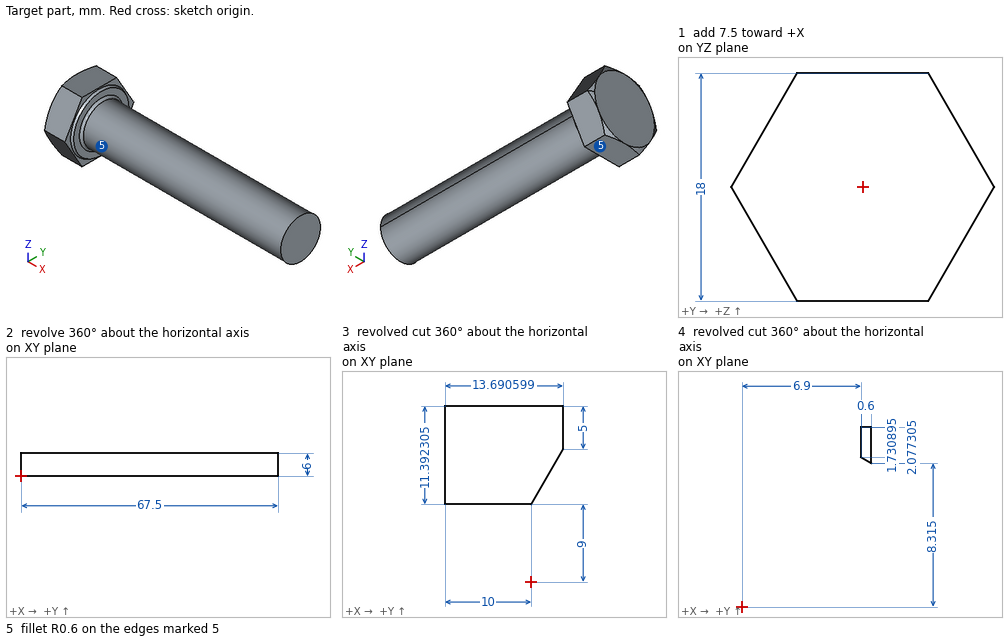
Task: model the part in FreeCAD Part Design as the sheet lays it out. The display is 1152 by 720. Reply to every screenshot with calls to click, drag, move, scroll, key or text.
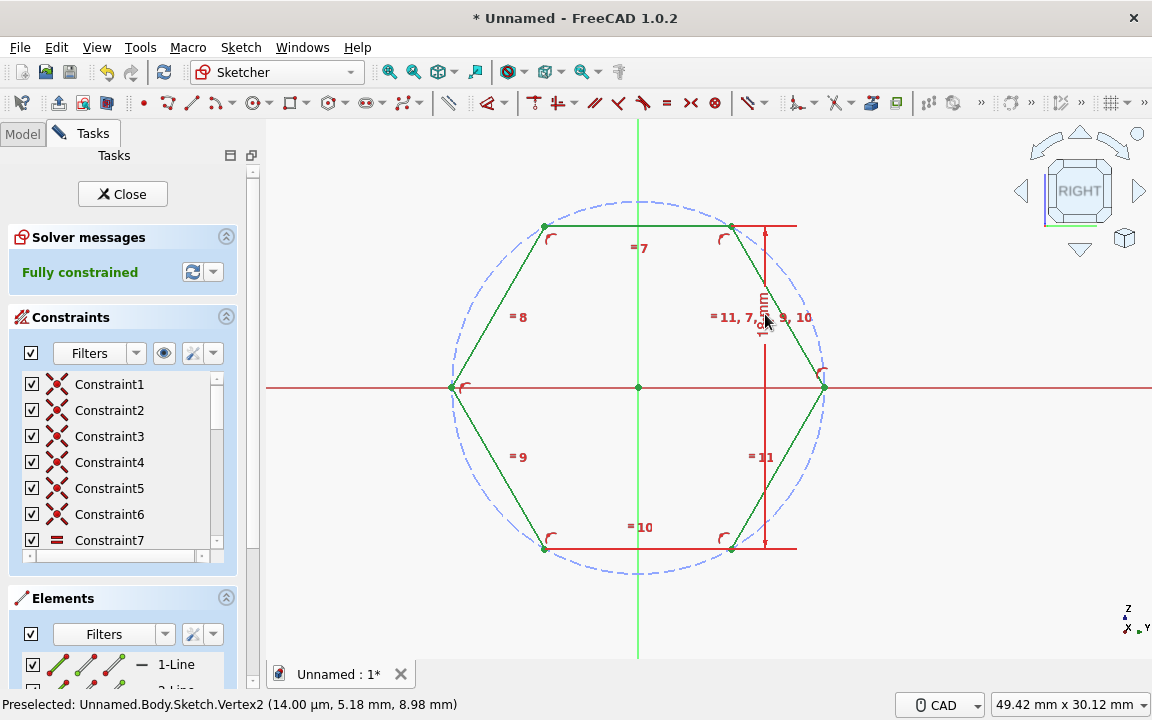
click(123, 194)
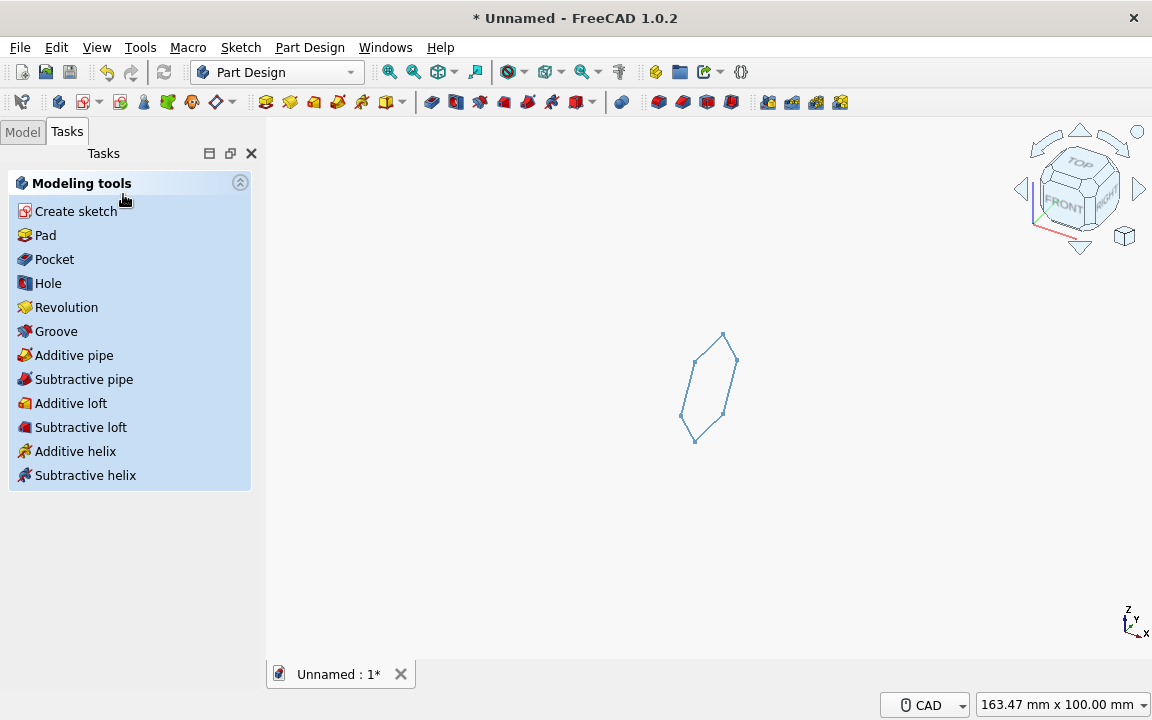
click(266, 102)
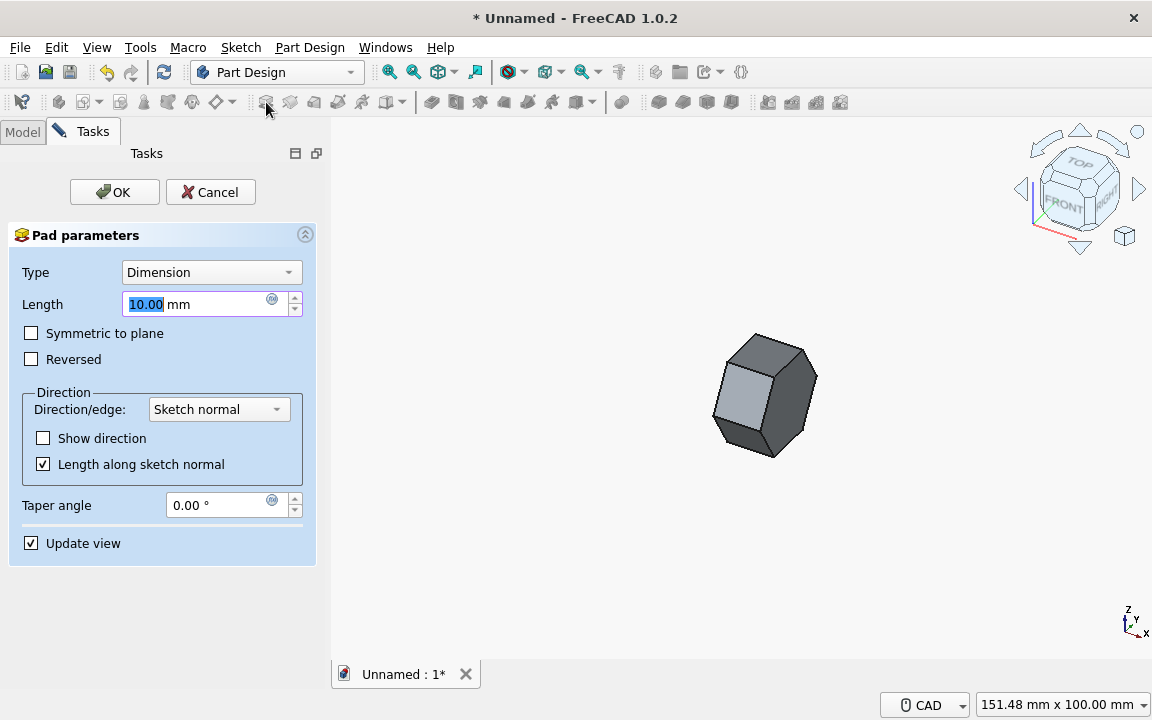
text(7.5)
key(Tab)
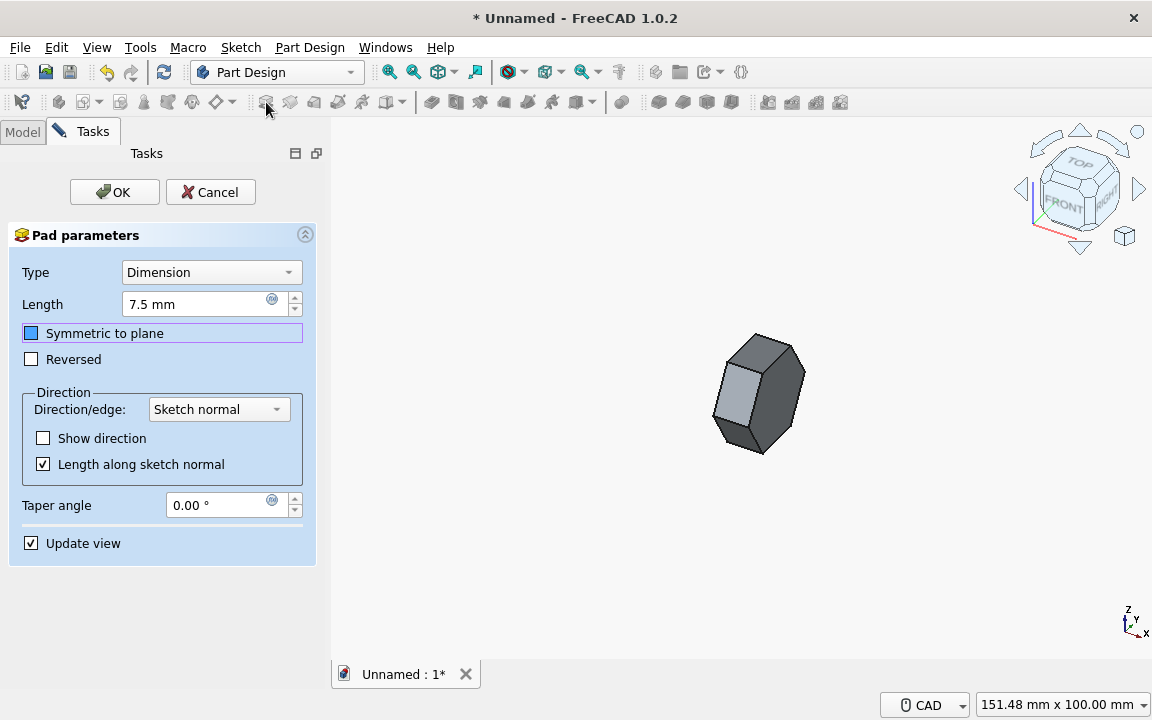
click(115, 192)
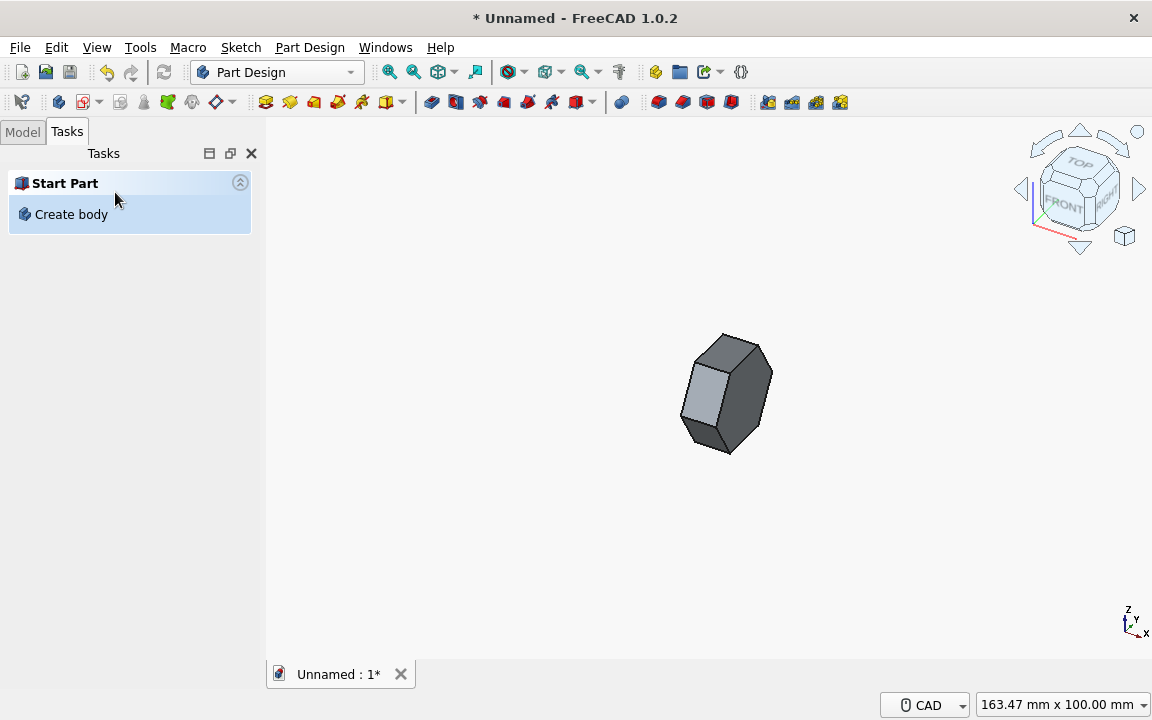
click(390, 72)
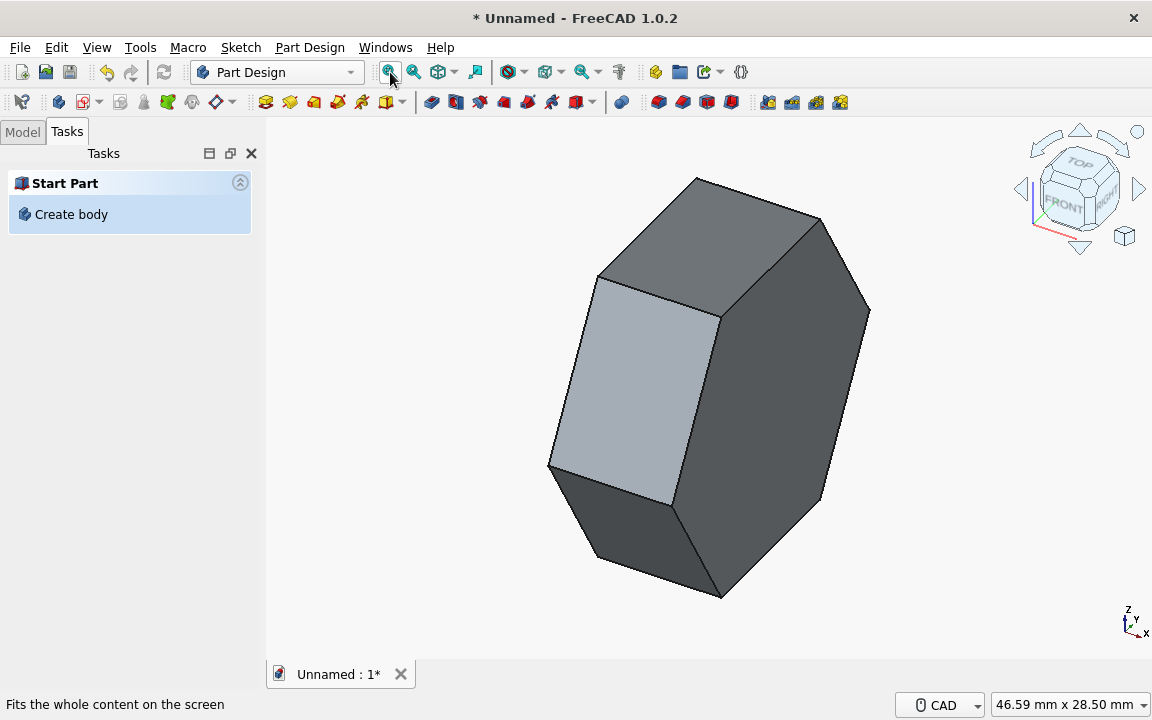
click(84, 102)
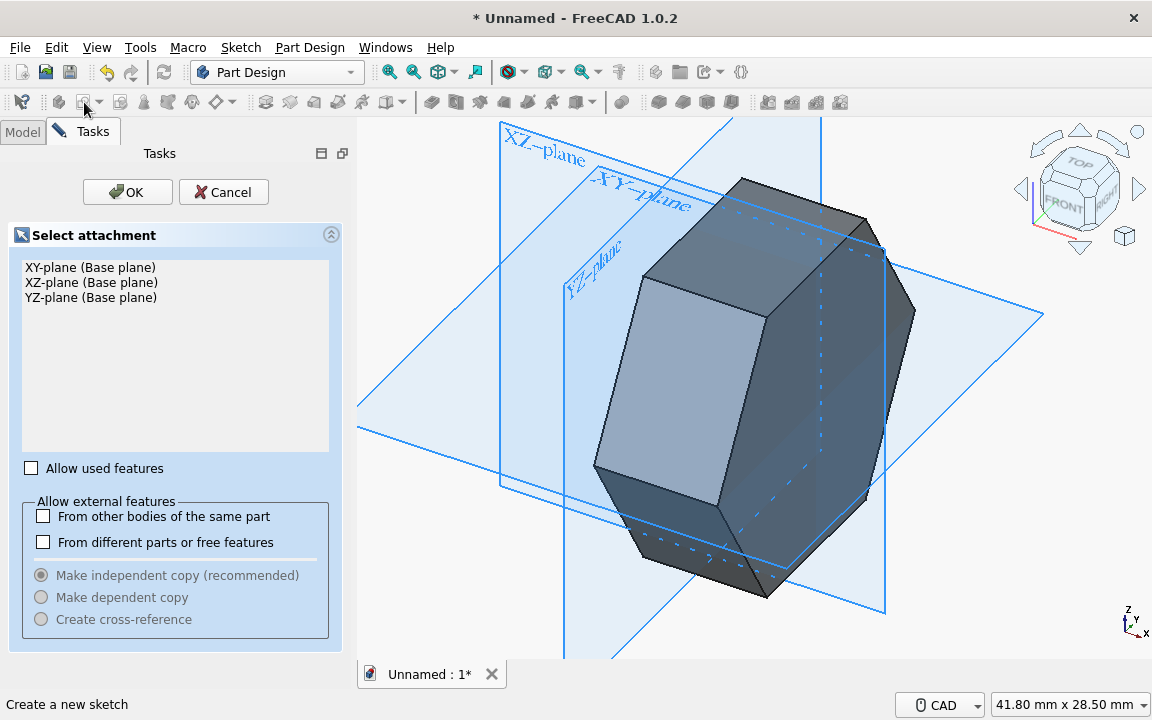
click(82, 268)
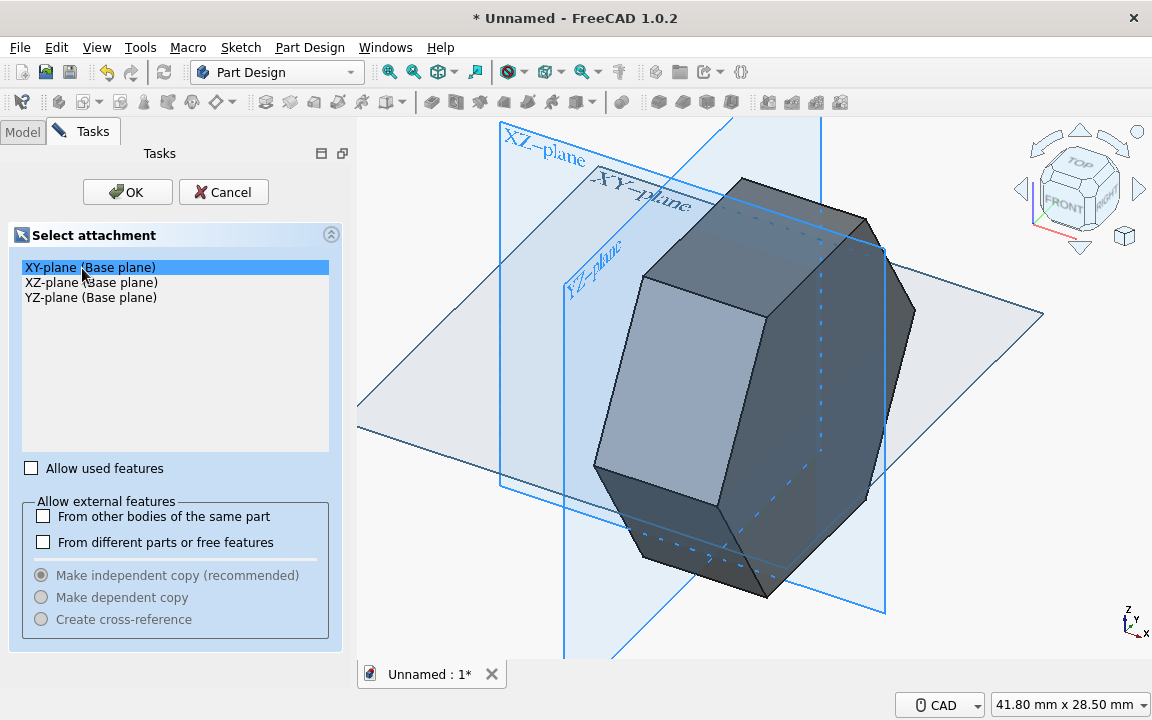
click(128, 192)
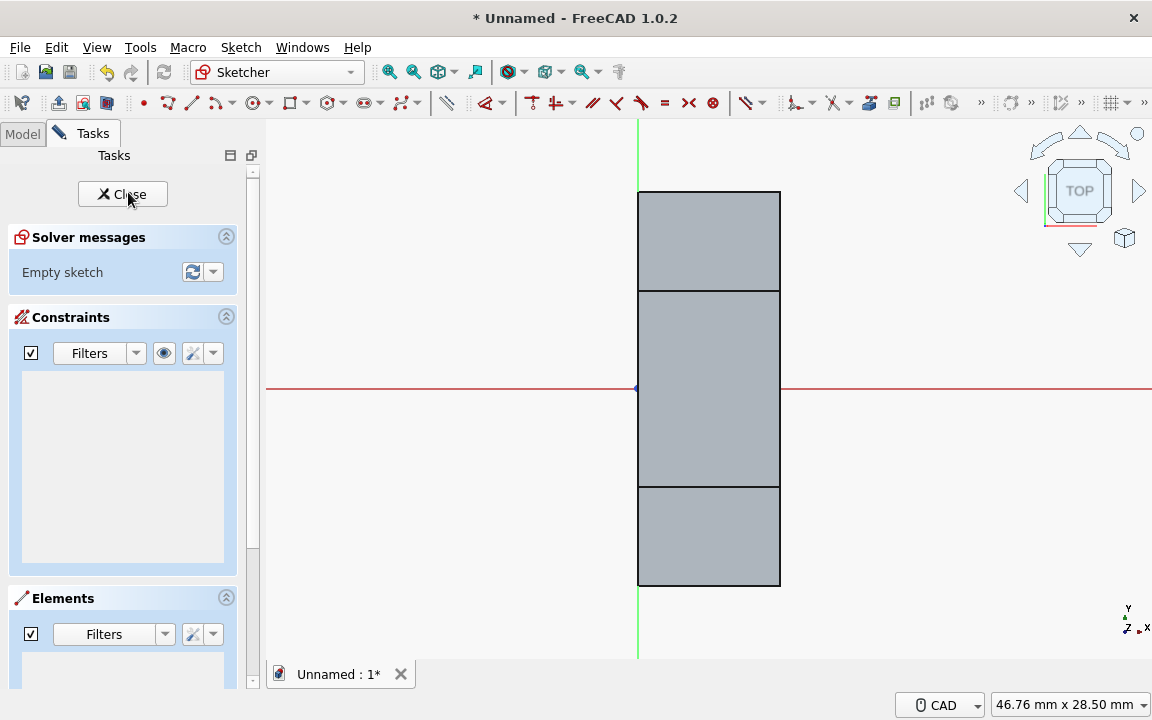
click(108, 104)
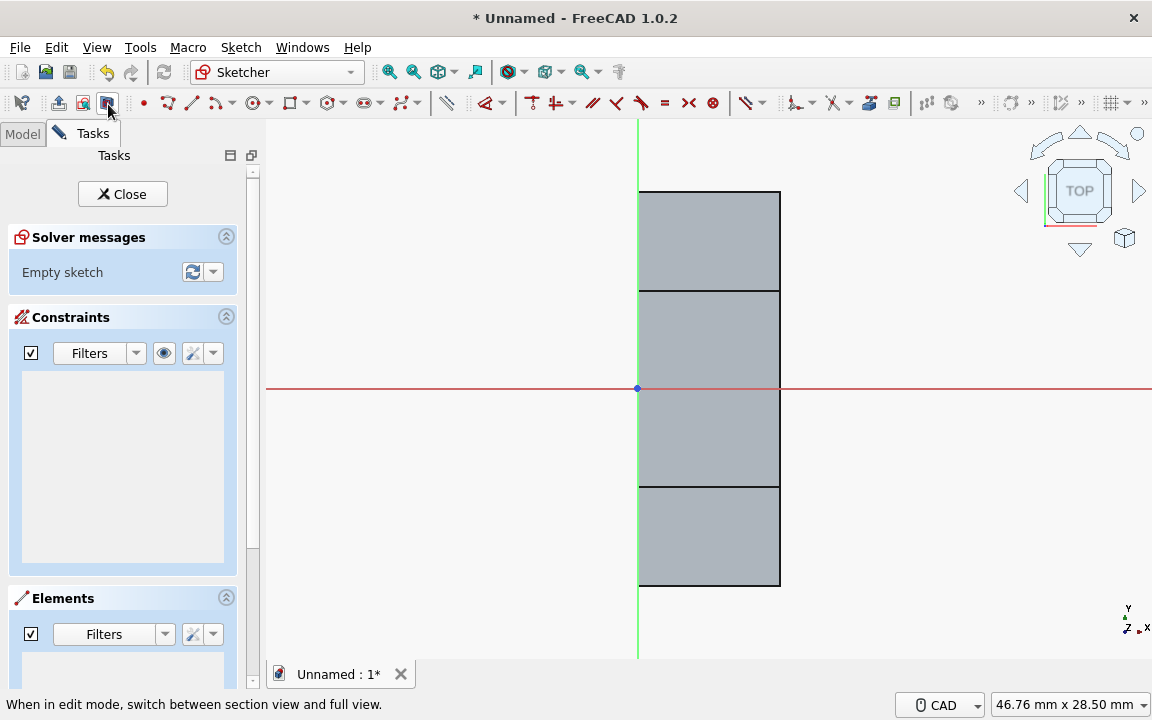
scroll(294, 422, down, 5)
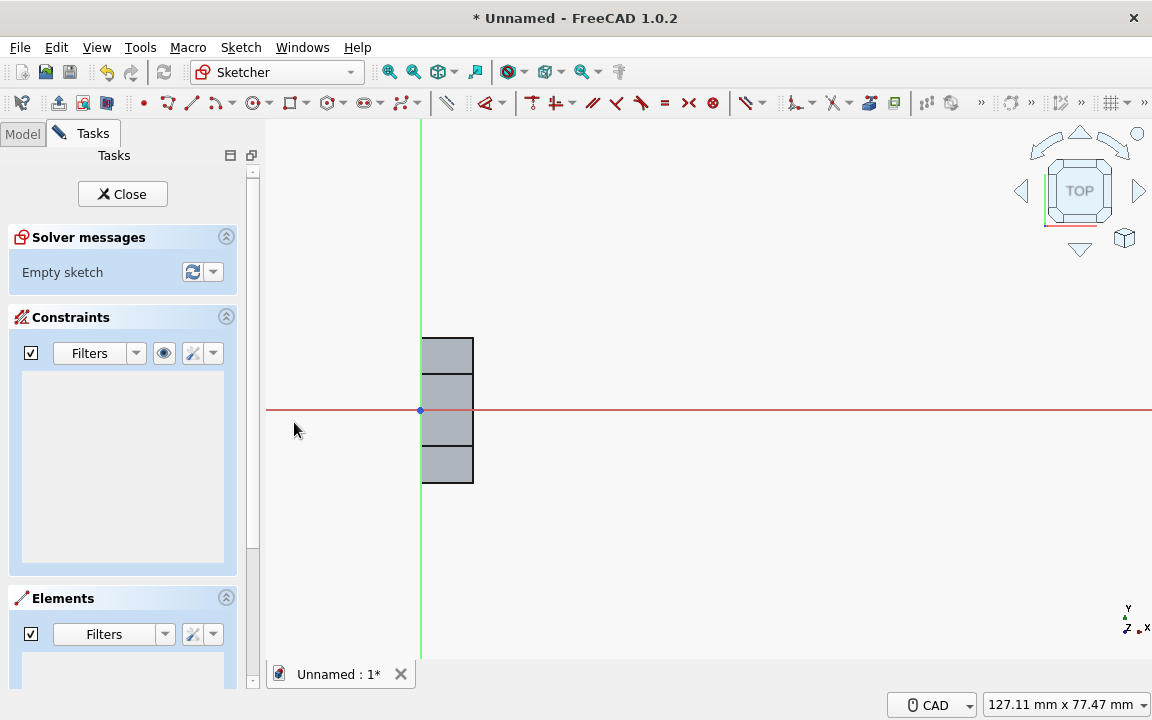
click(290, 104)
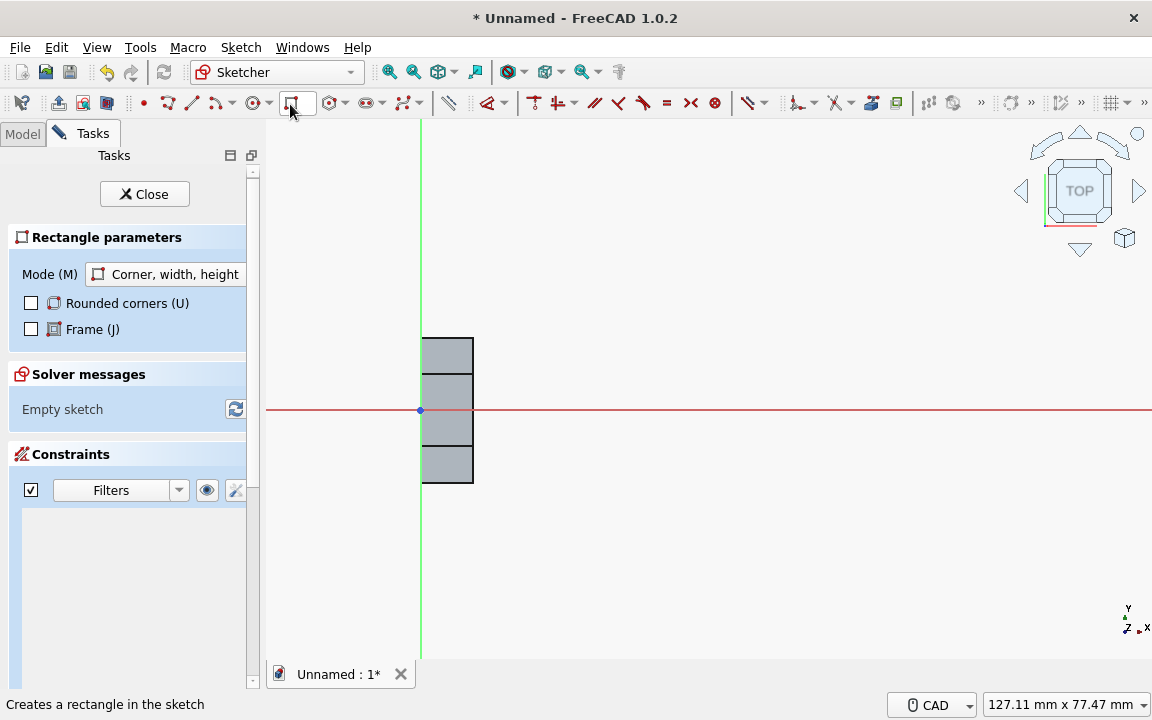
click(421, 410)
move(891, 368)